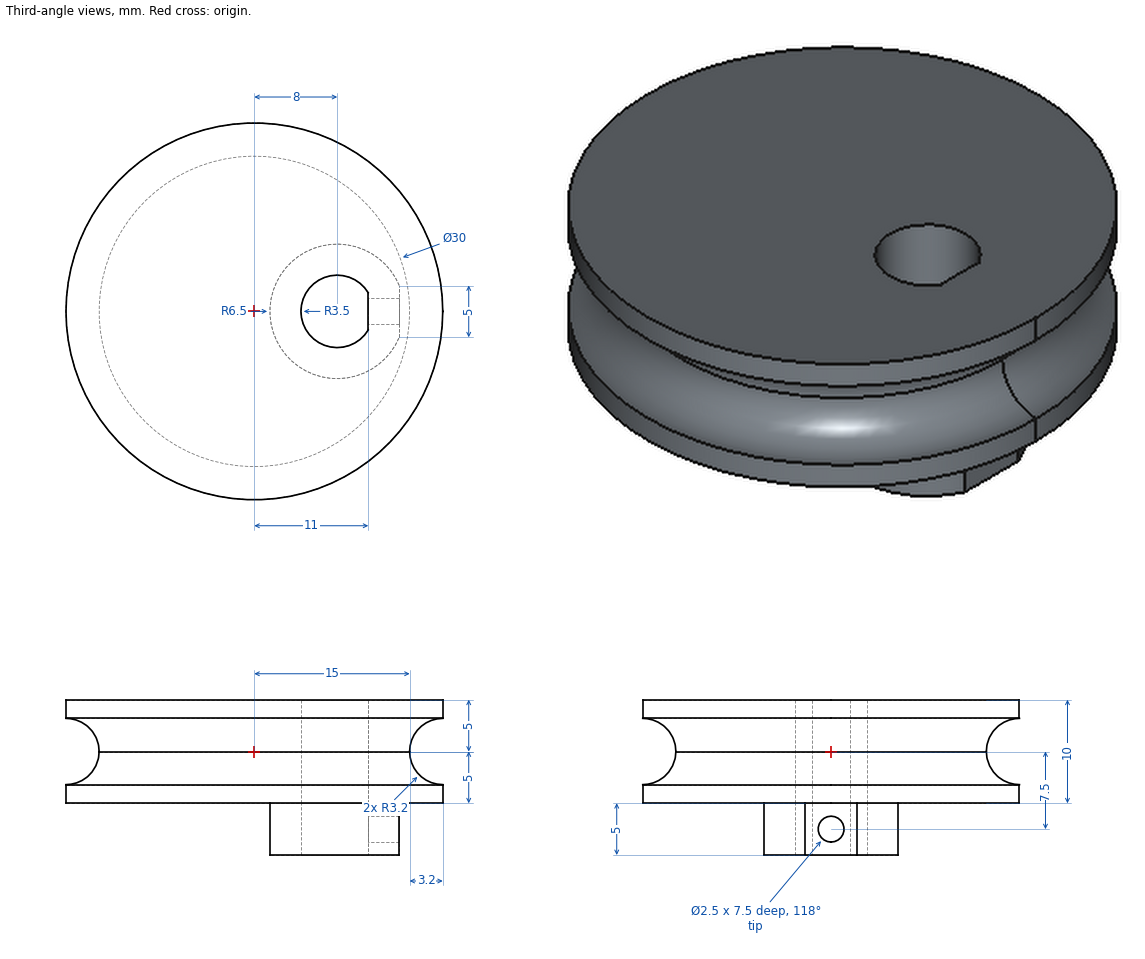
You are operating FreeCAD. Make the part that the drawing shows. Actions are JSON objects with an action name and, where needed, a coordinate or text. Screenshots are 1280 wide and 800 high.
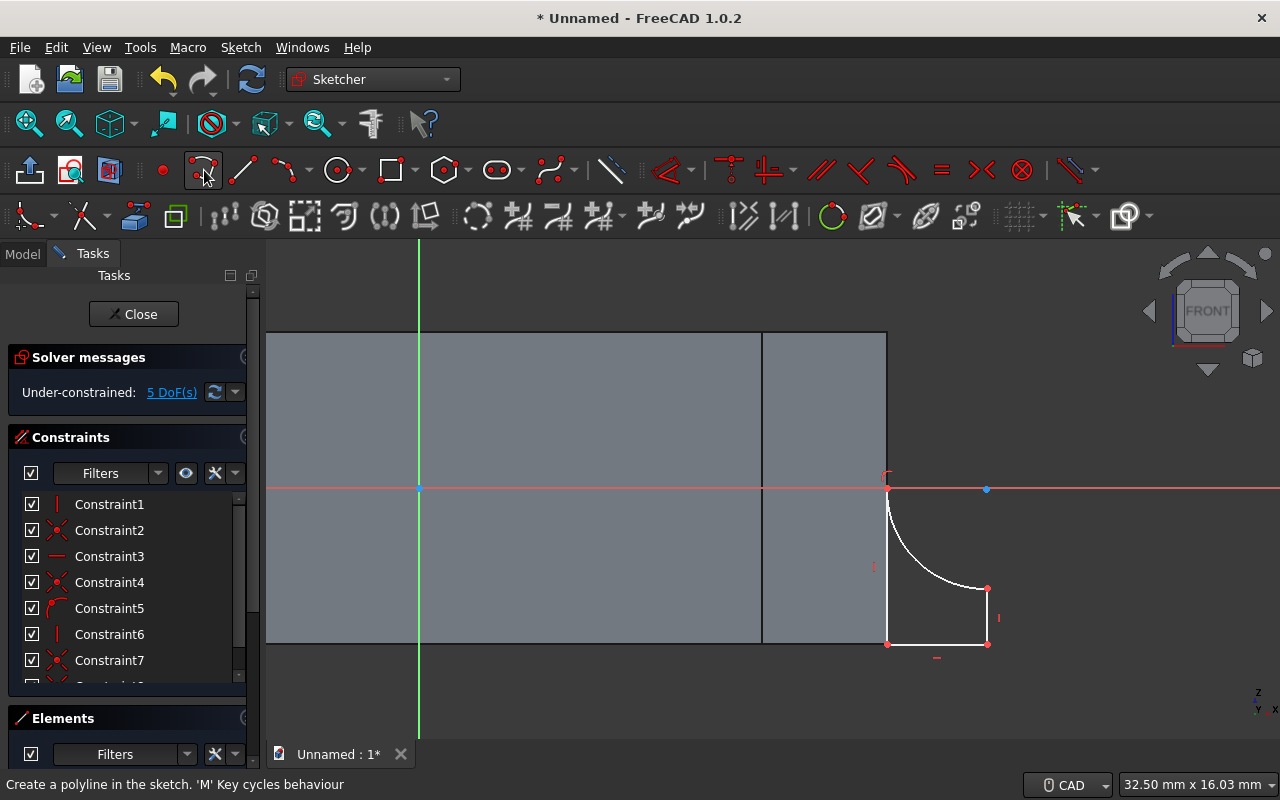
{"action": "left_click", "coordinate": [887, 488]}
{"action": "left_click", "coordinate": [887, 332]}
{"action": "left_click", "coordinate": [987, 332]}
{"action": "left_click", "coordinate": [987, 388]}
{"action": "right_click", "coordinate": [987, 388]}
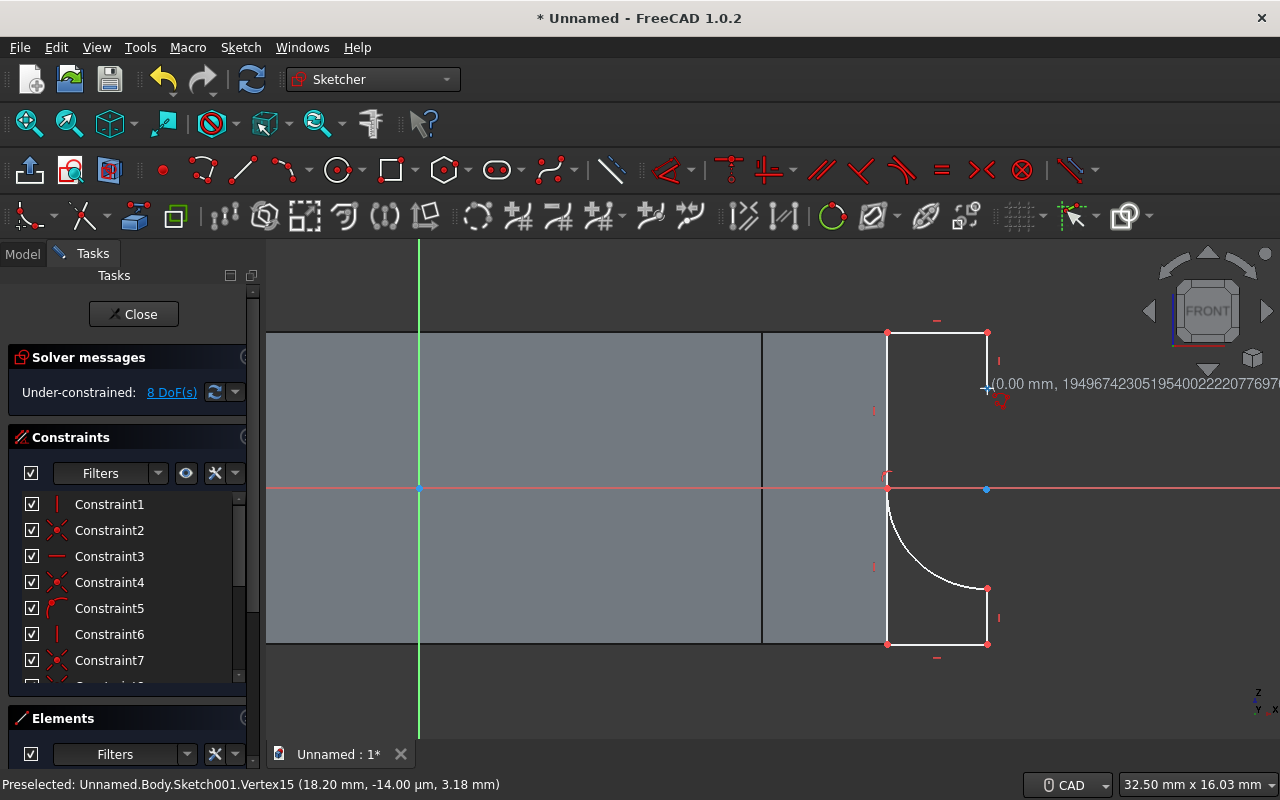
{"action": "left_click", "coordinate": [284, 170]}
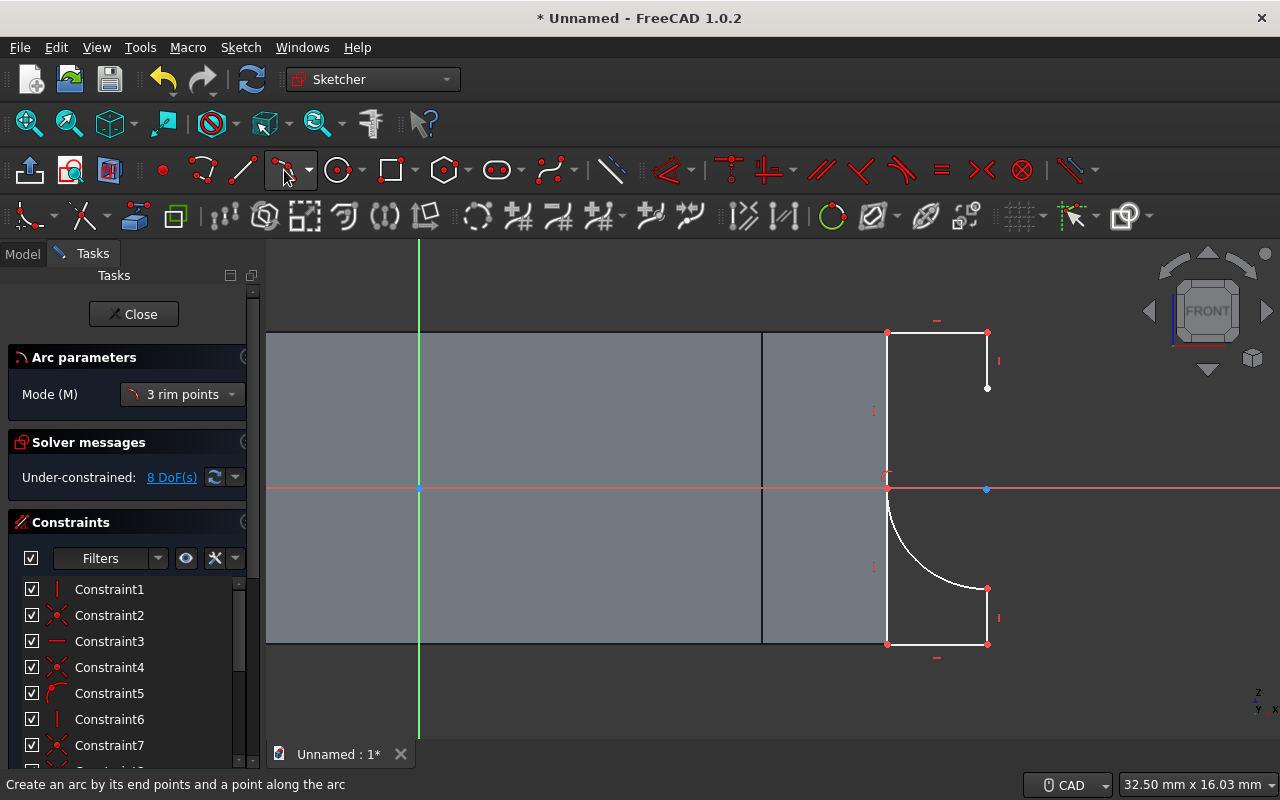
{"action": "left_click", "coordinate": [987, 389]}
{"action": "left_click", "coordinate": [887, 488]}
{"action": "left_click", "coordinate": [916, 418]}
{"action": "key", "text": "Escape"}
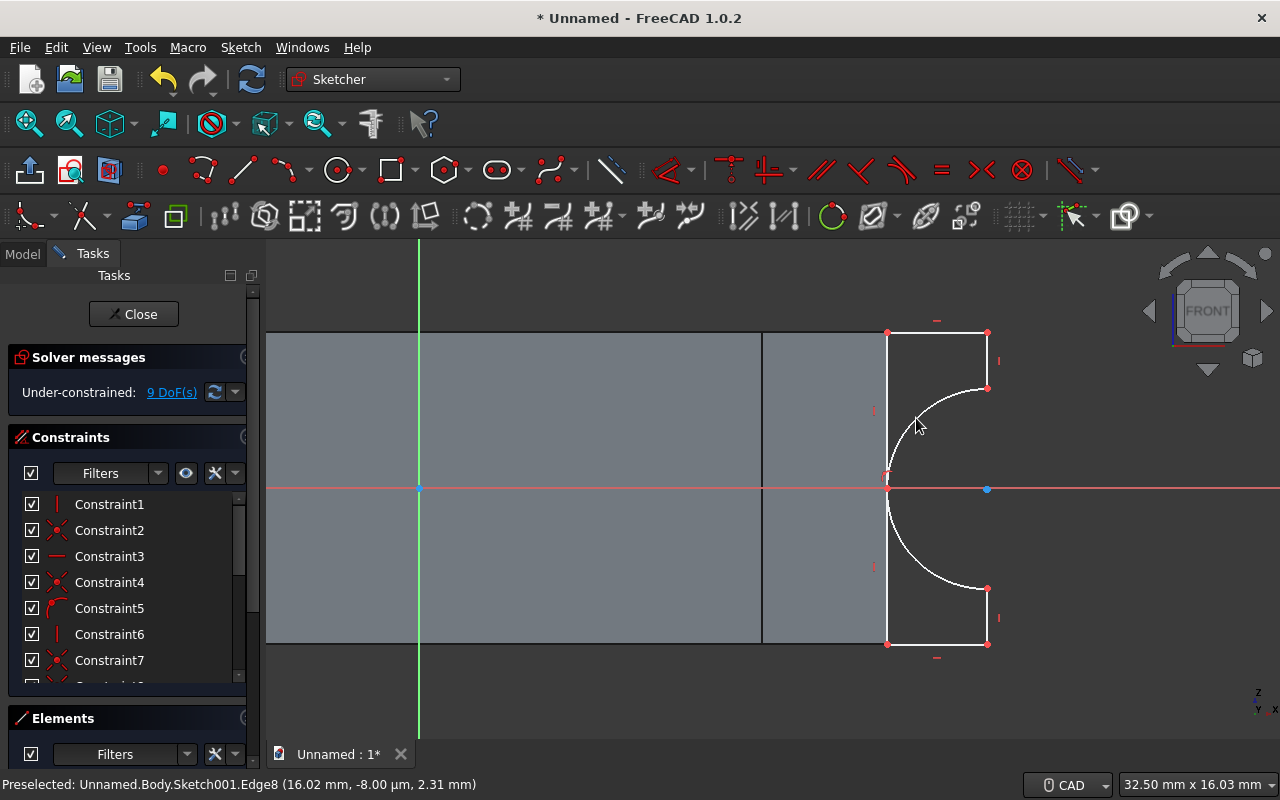
{"action": "left_click", "coordinate": [887, 598]}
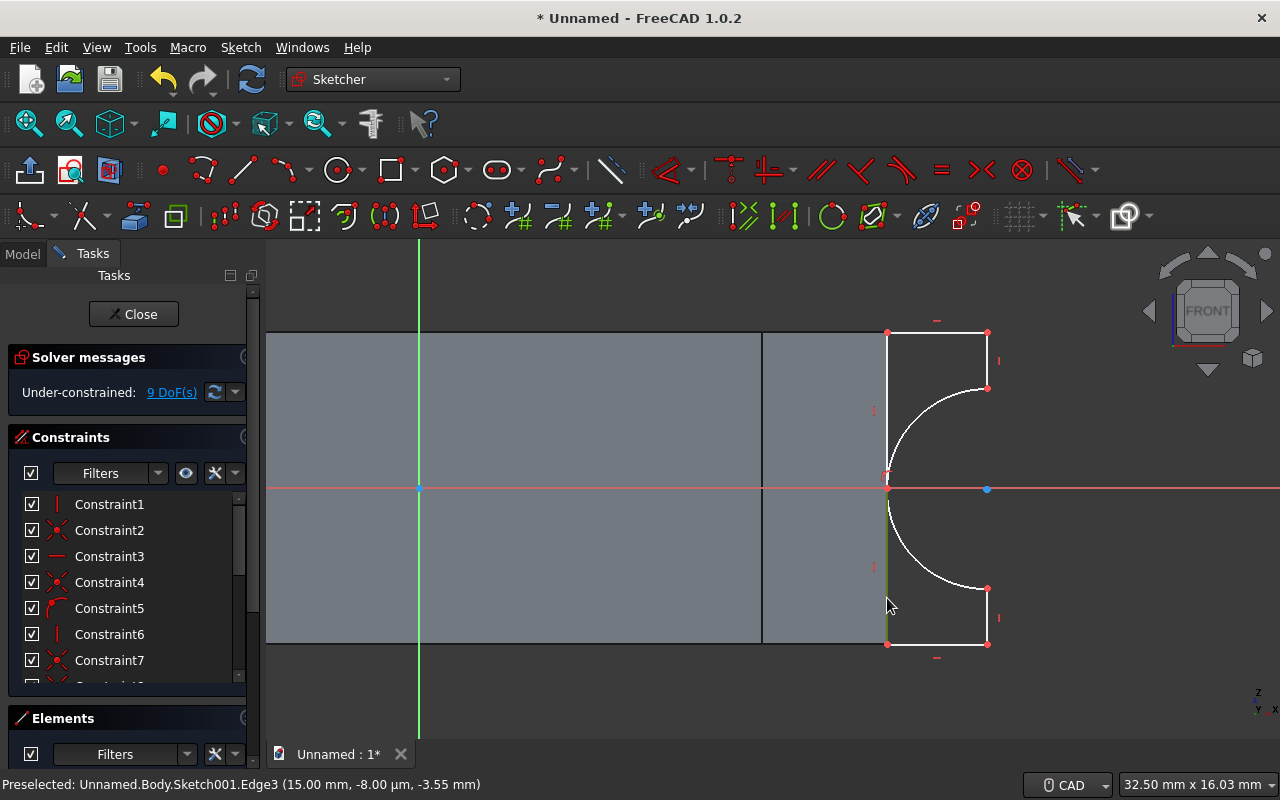
{"action": "scroll", "coordinate": [897, 534], "scroll_direction": "up", "scroll_amount": 2}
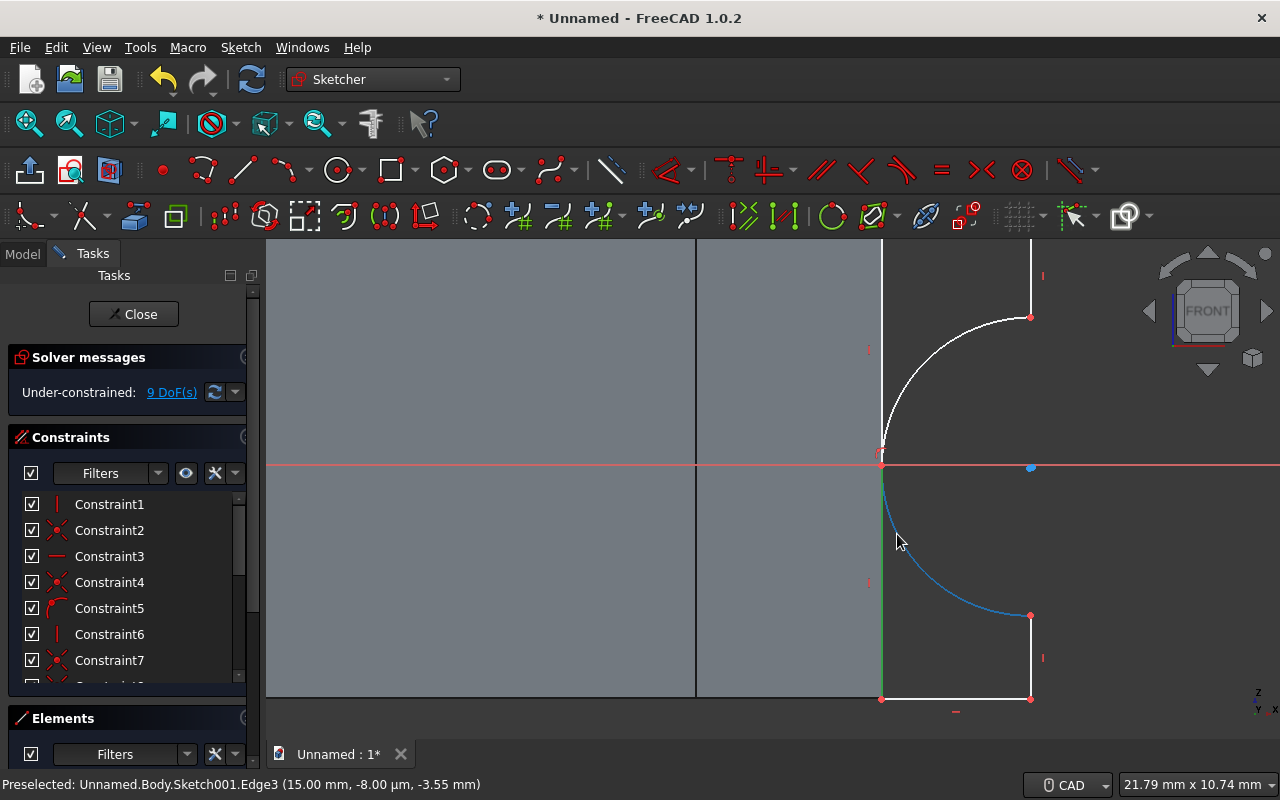
{"action": "left_click", "coordinate": [897, 534]}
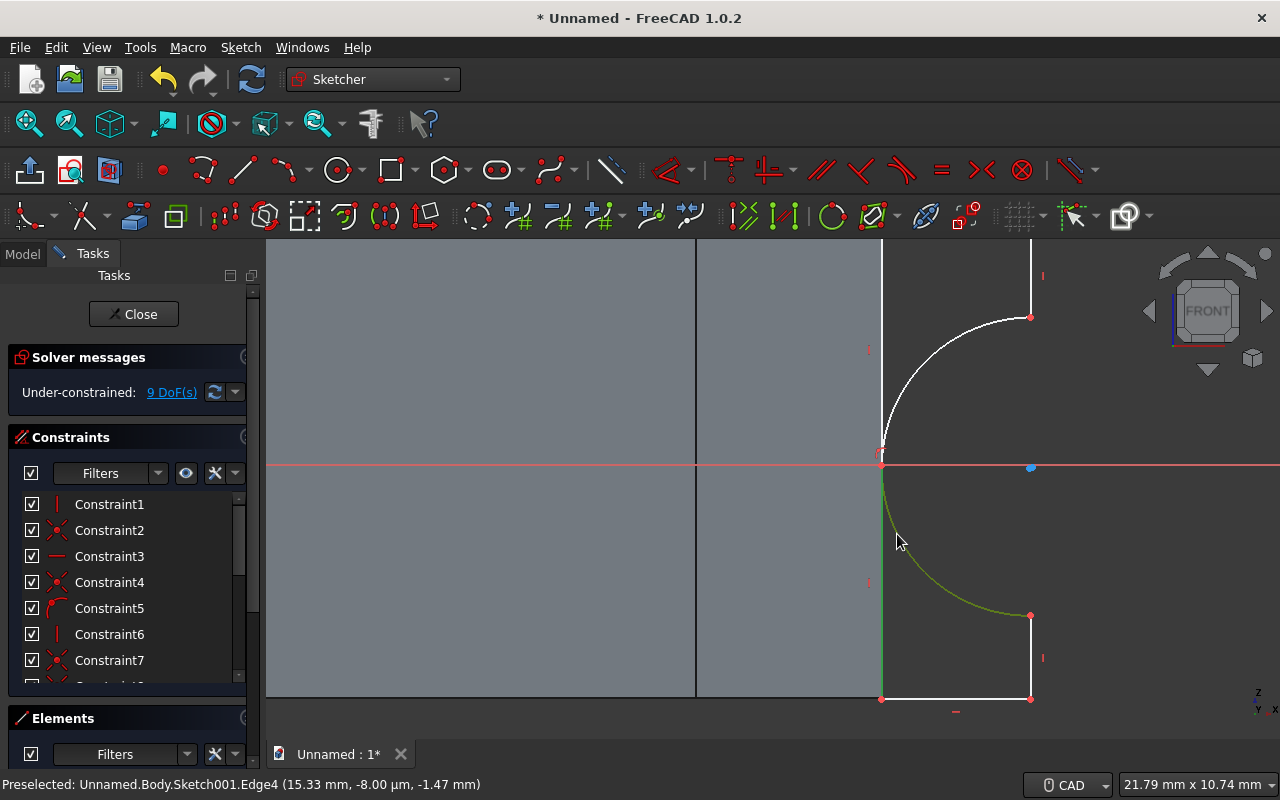
{"action": "left_click", "coordinate": [902, 170]}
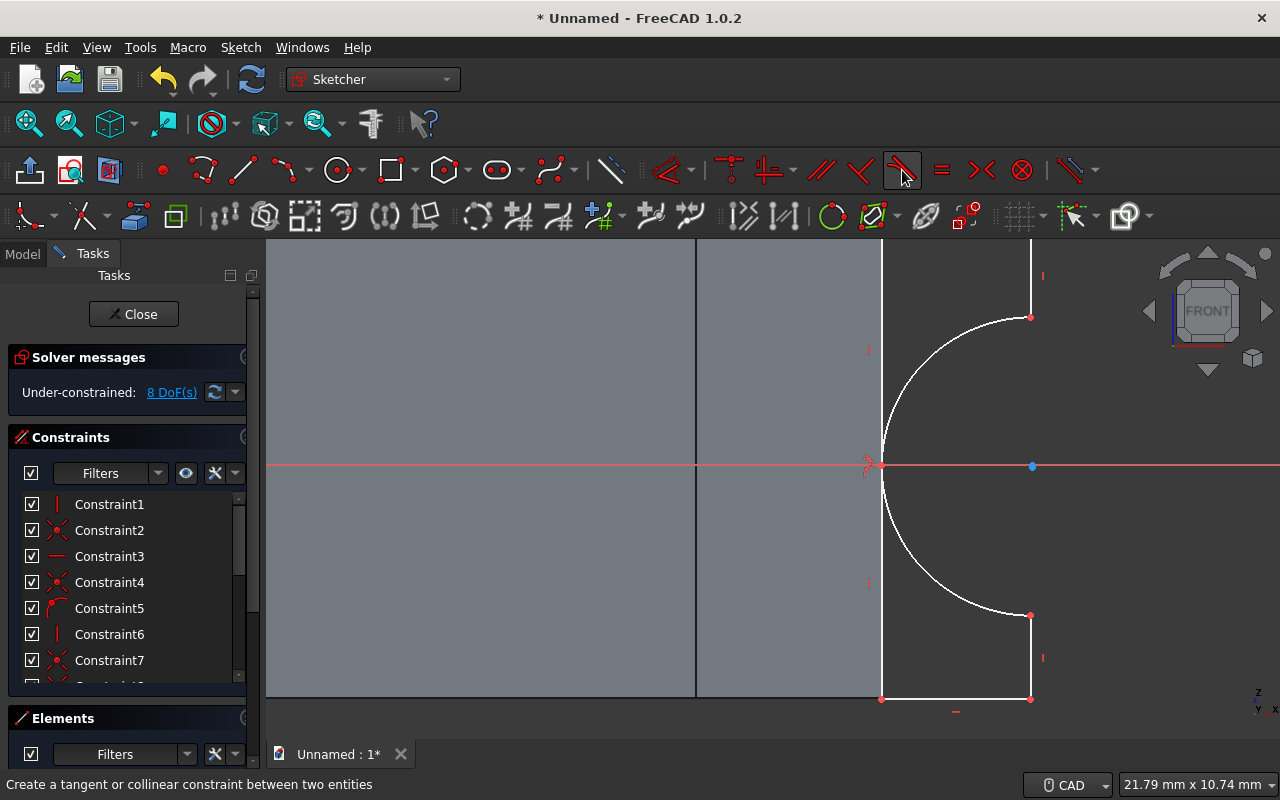
{"action": "left_click", "coordinate": [882, 629]}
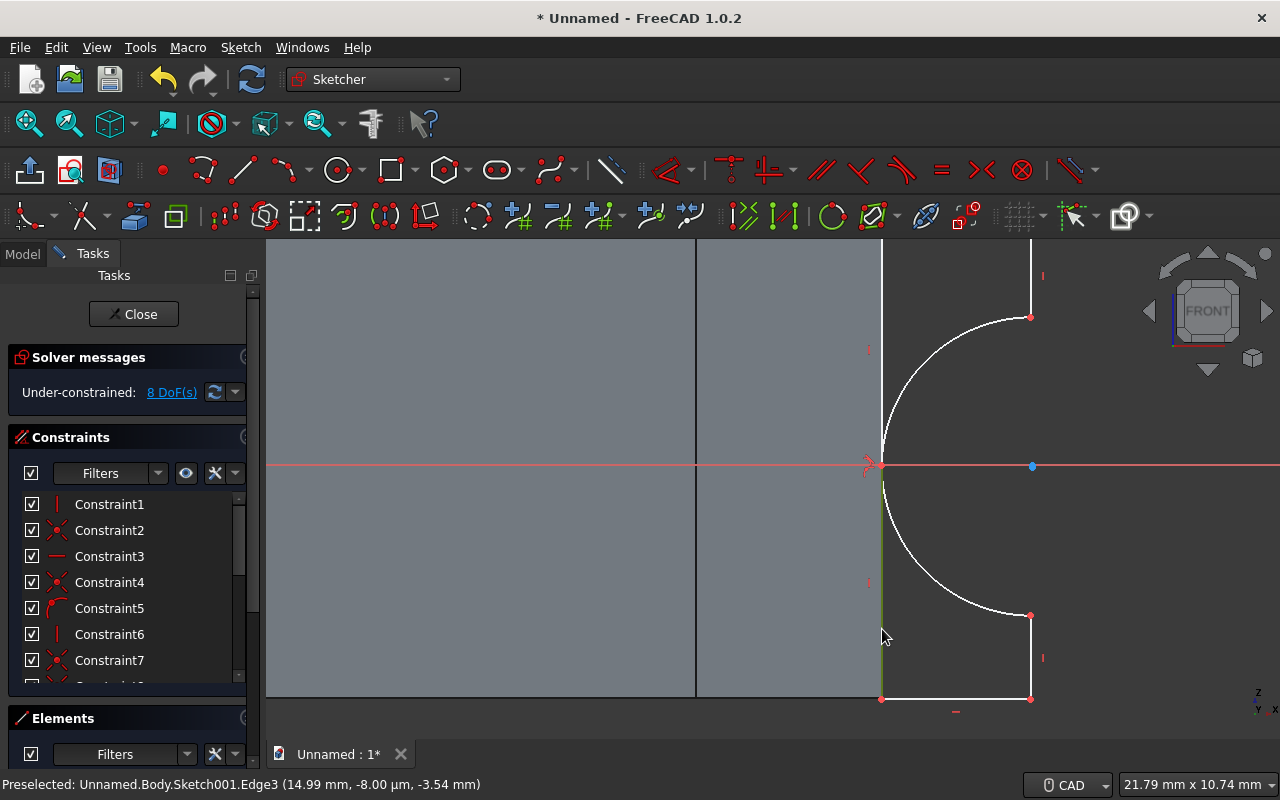
{"action": "left_click", "coordinate": [964, 334]}